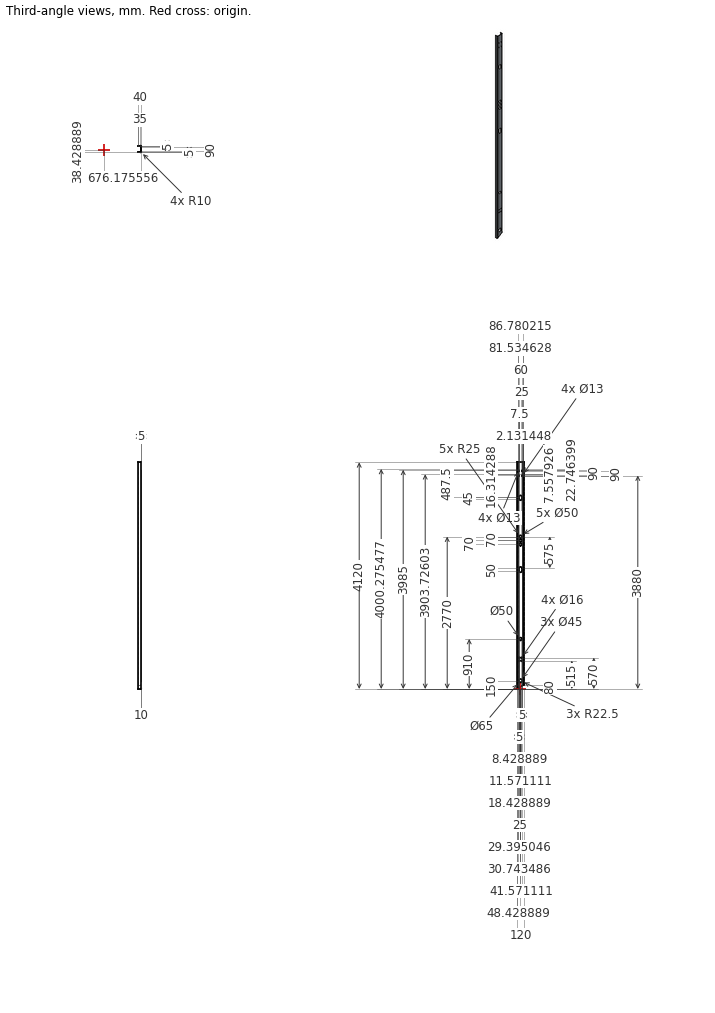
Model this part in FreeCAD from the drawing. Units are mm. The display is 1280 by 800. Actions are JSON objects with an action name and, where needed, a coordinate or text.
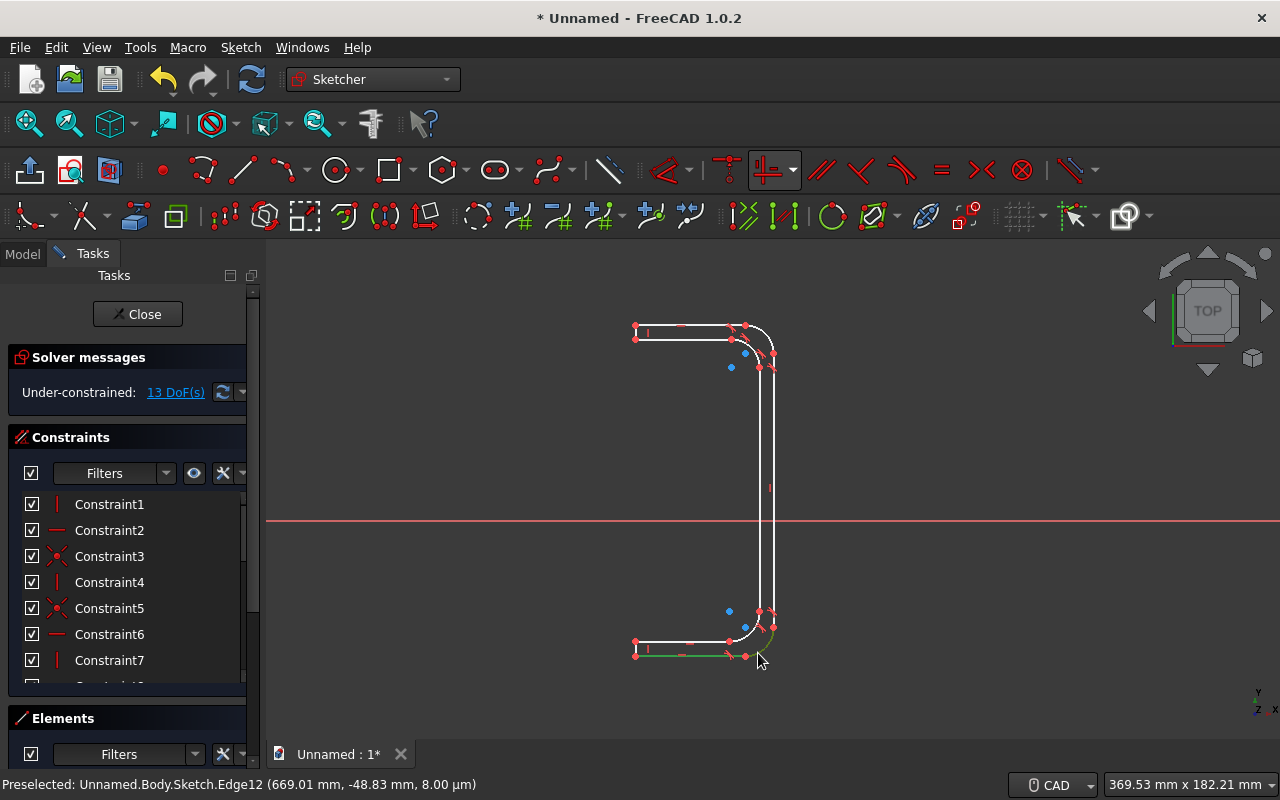
{"action": "key", "text": "t"}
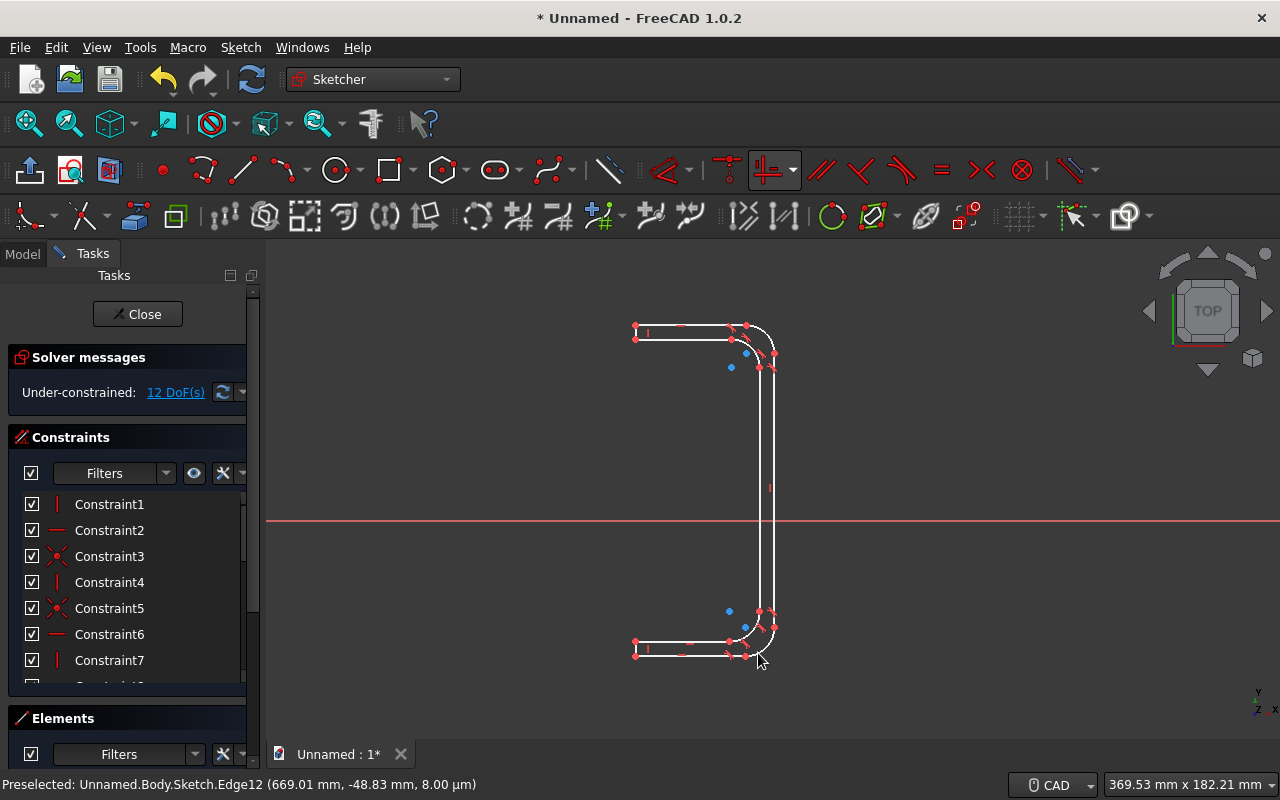
{"action": "left_click", "coordinate": [771, 341]}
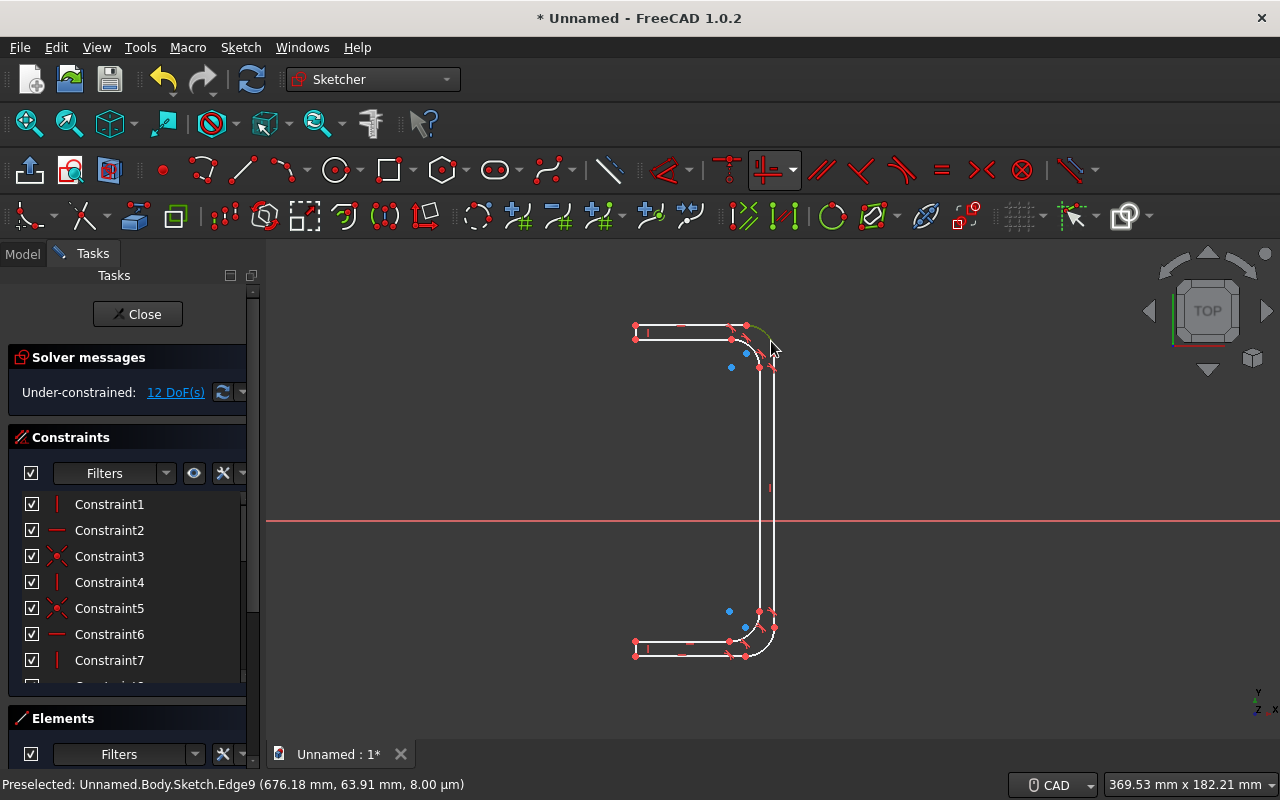
{"action": "left_click", "coordinate": [744, 343]}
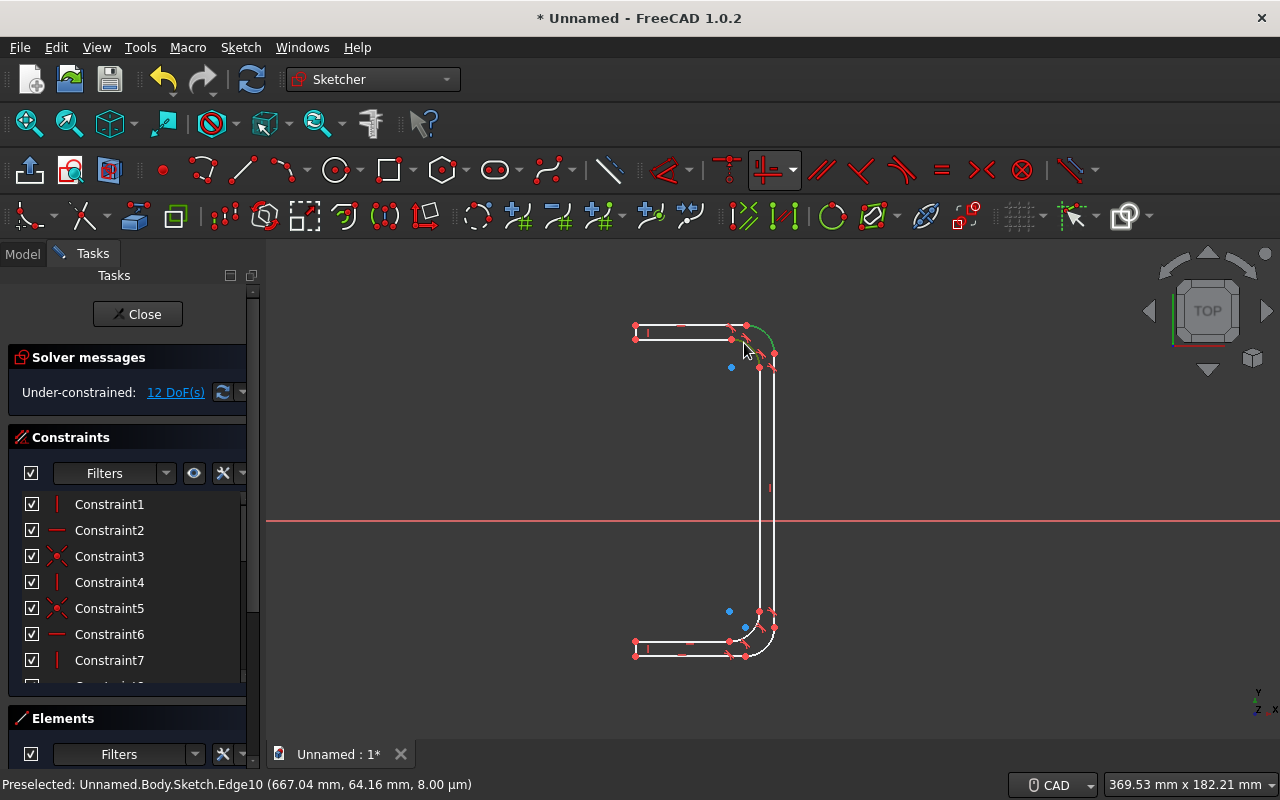
{"action": "left_click", "coordinate": [751, 633]}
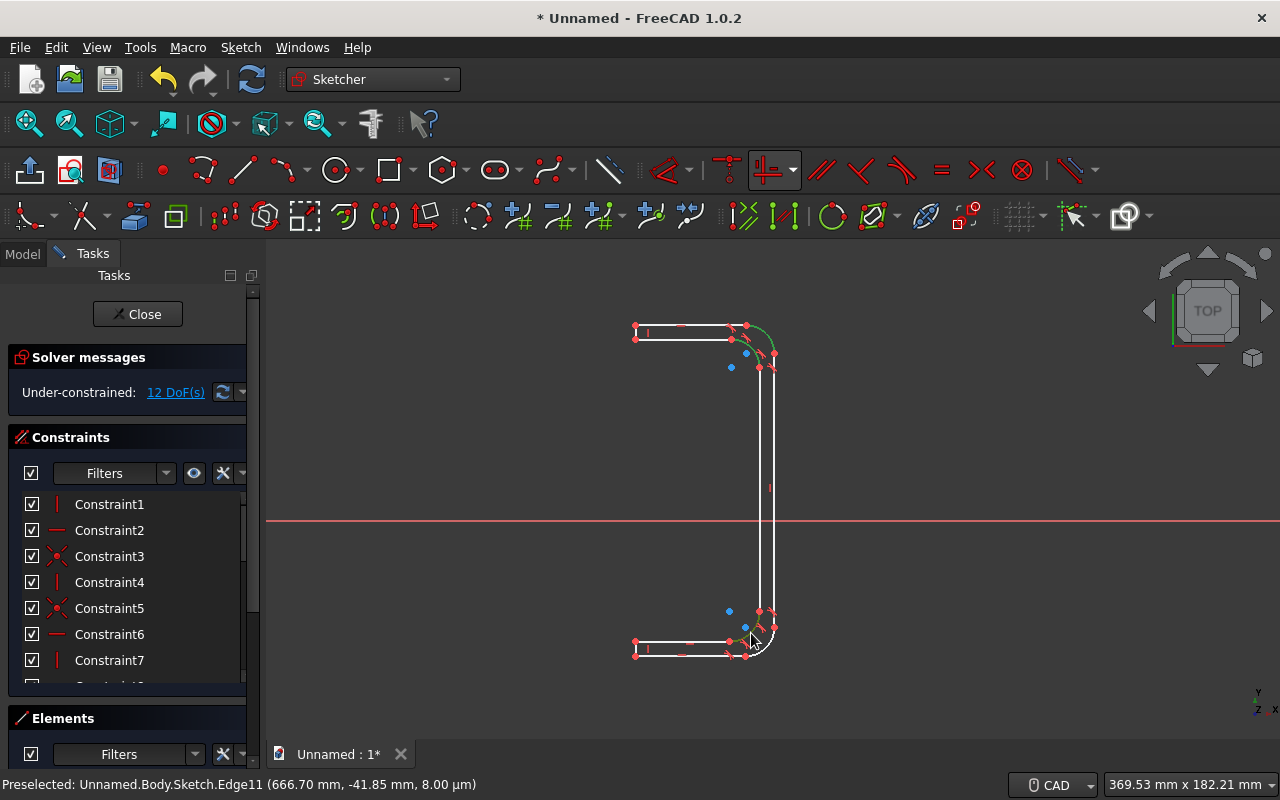
{"action": "left_click", "coordinate": [759, 653]}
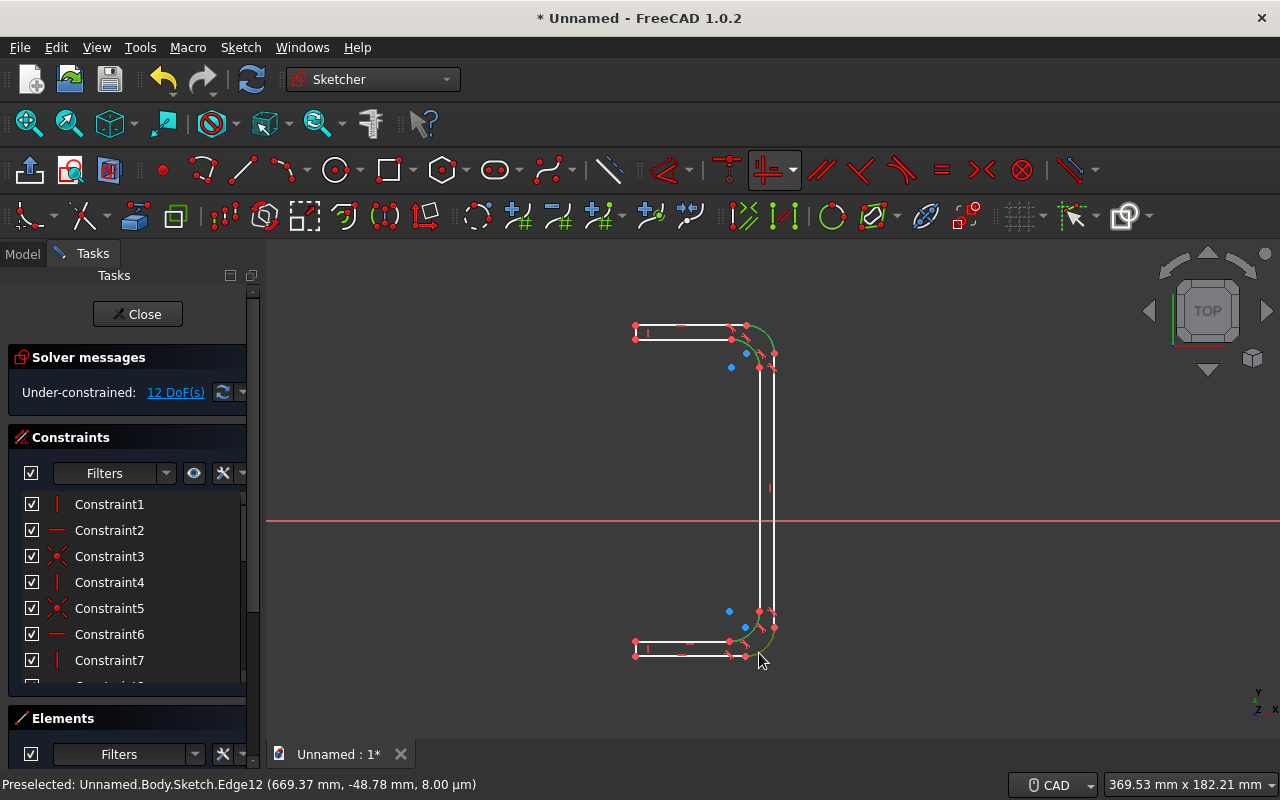
{"action": "key", "text": "e"}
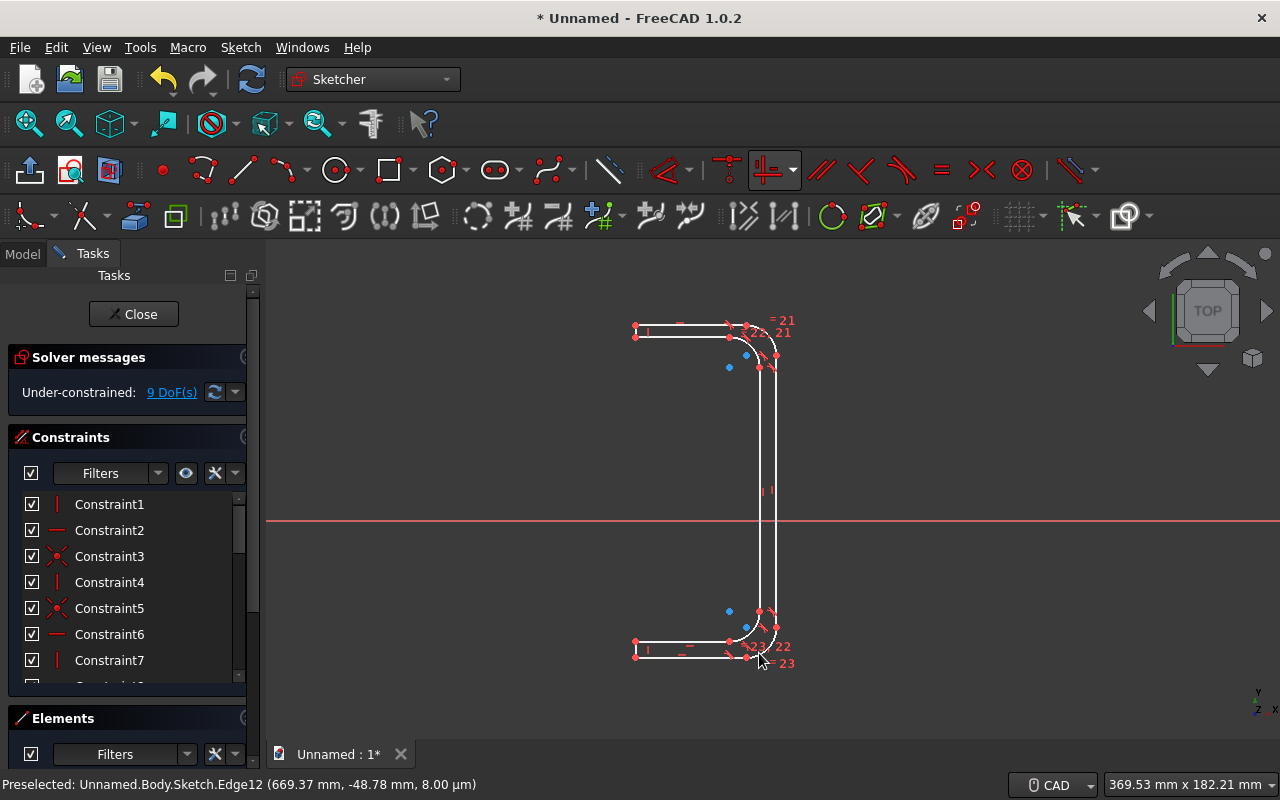
{"action": "key", "text": "d"}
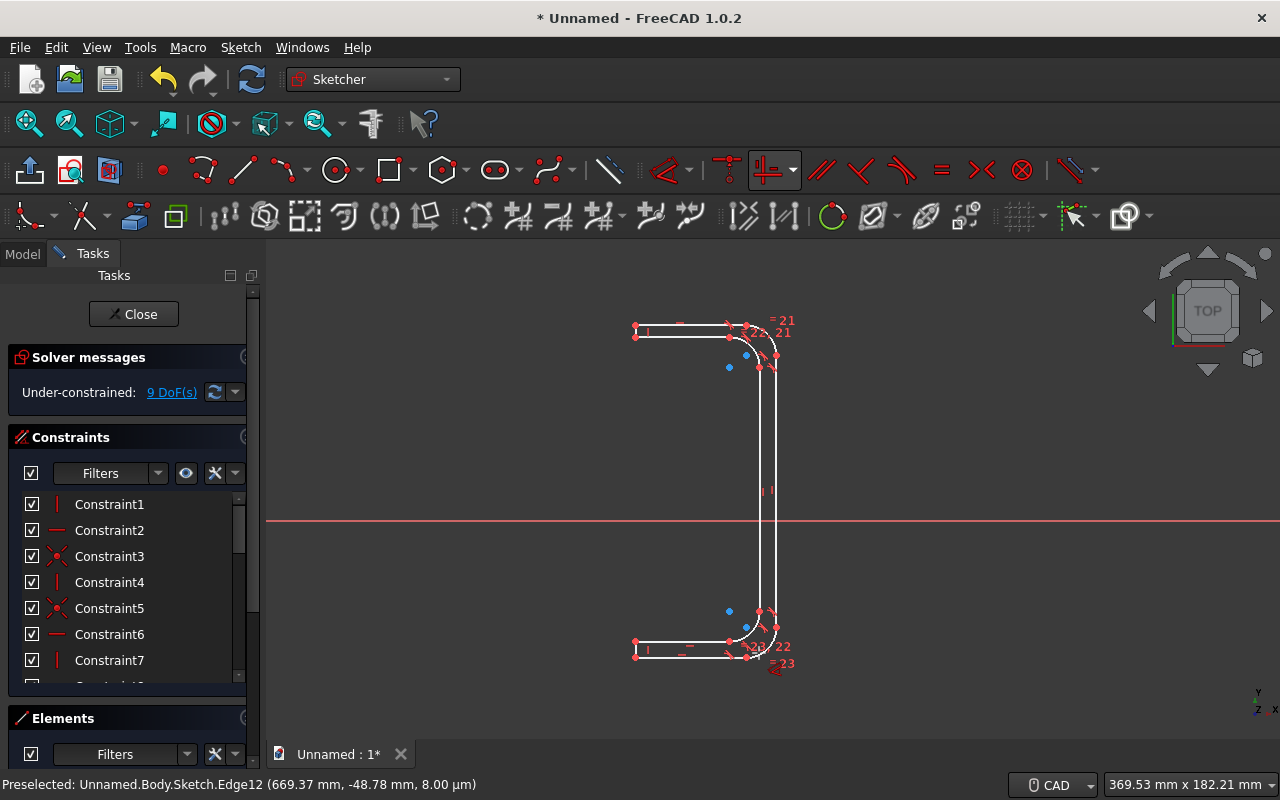
{"action": "scroll", "coordinate": [773, 342], "scroll_direction": "up", "scroll_amount": 2}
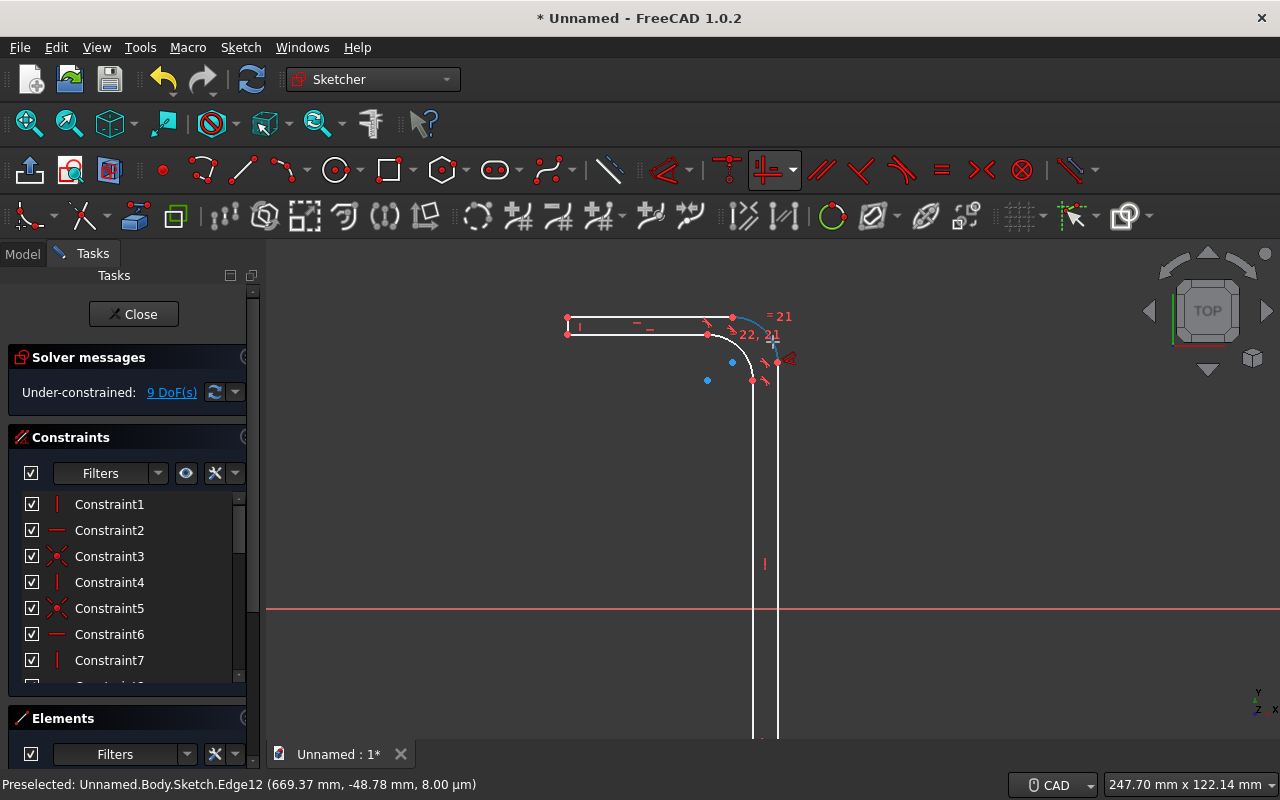
{"action": "left_click", "coordinate": [773, 342]}
{"action": "left_click", "coordinate": [802, 328]}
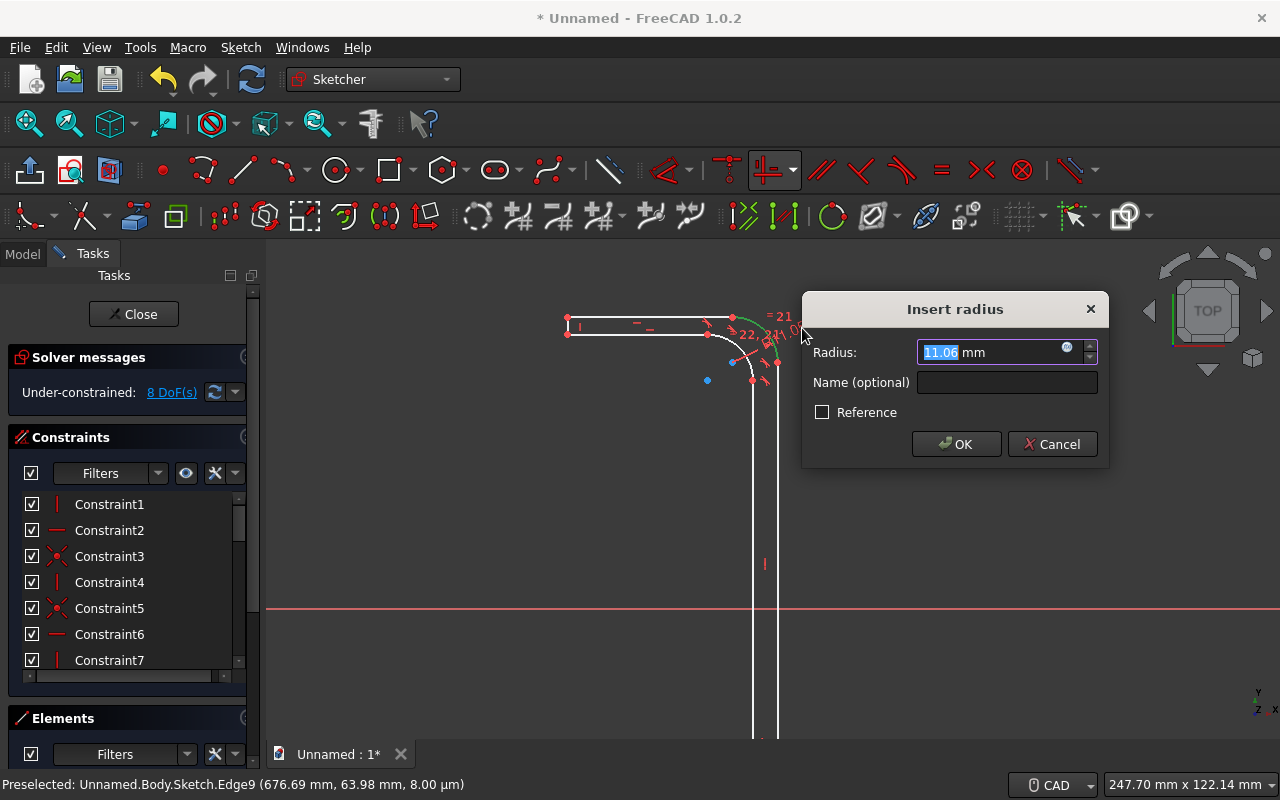
{"action": "type", "text": "10"}
{"action": "key", "text": "Return"}